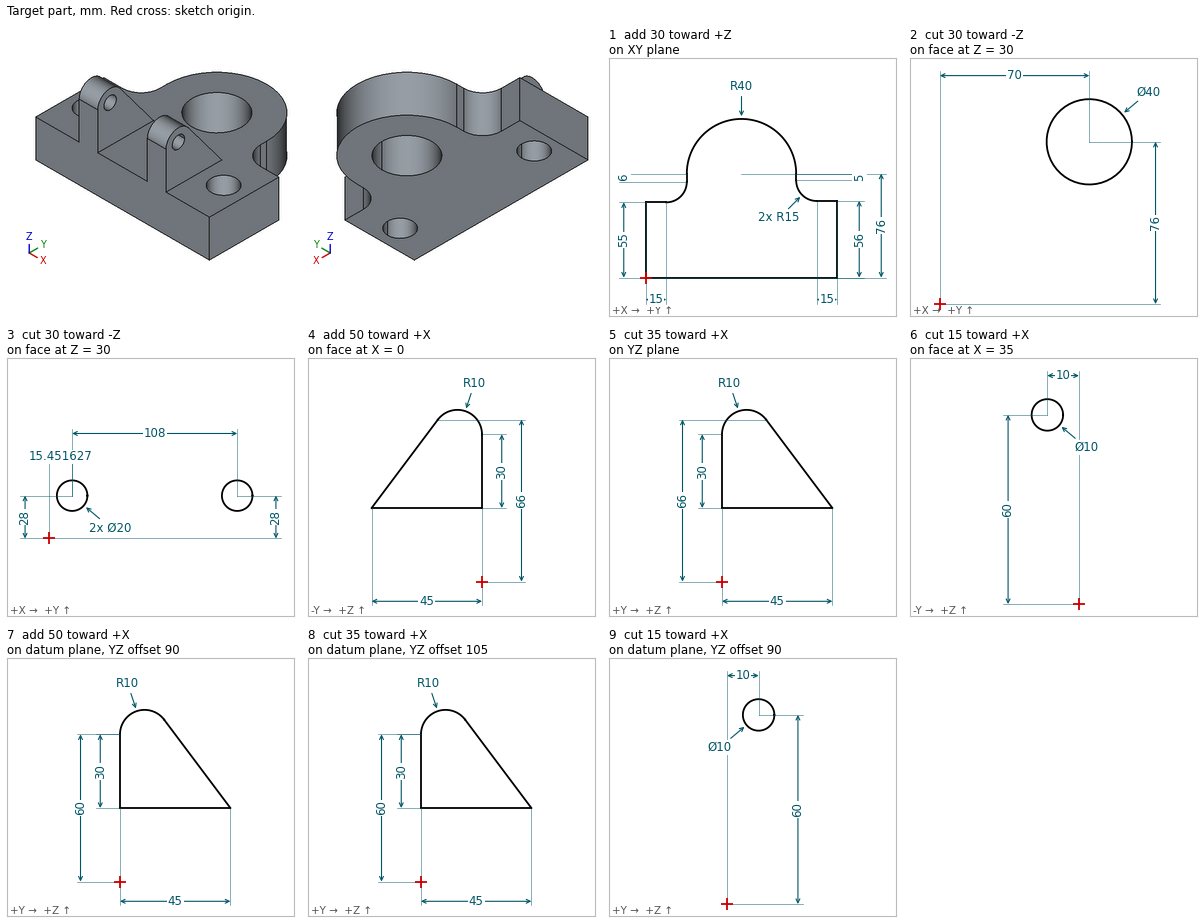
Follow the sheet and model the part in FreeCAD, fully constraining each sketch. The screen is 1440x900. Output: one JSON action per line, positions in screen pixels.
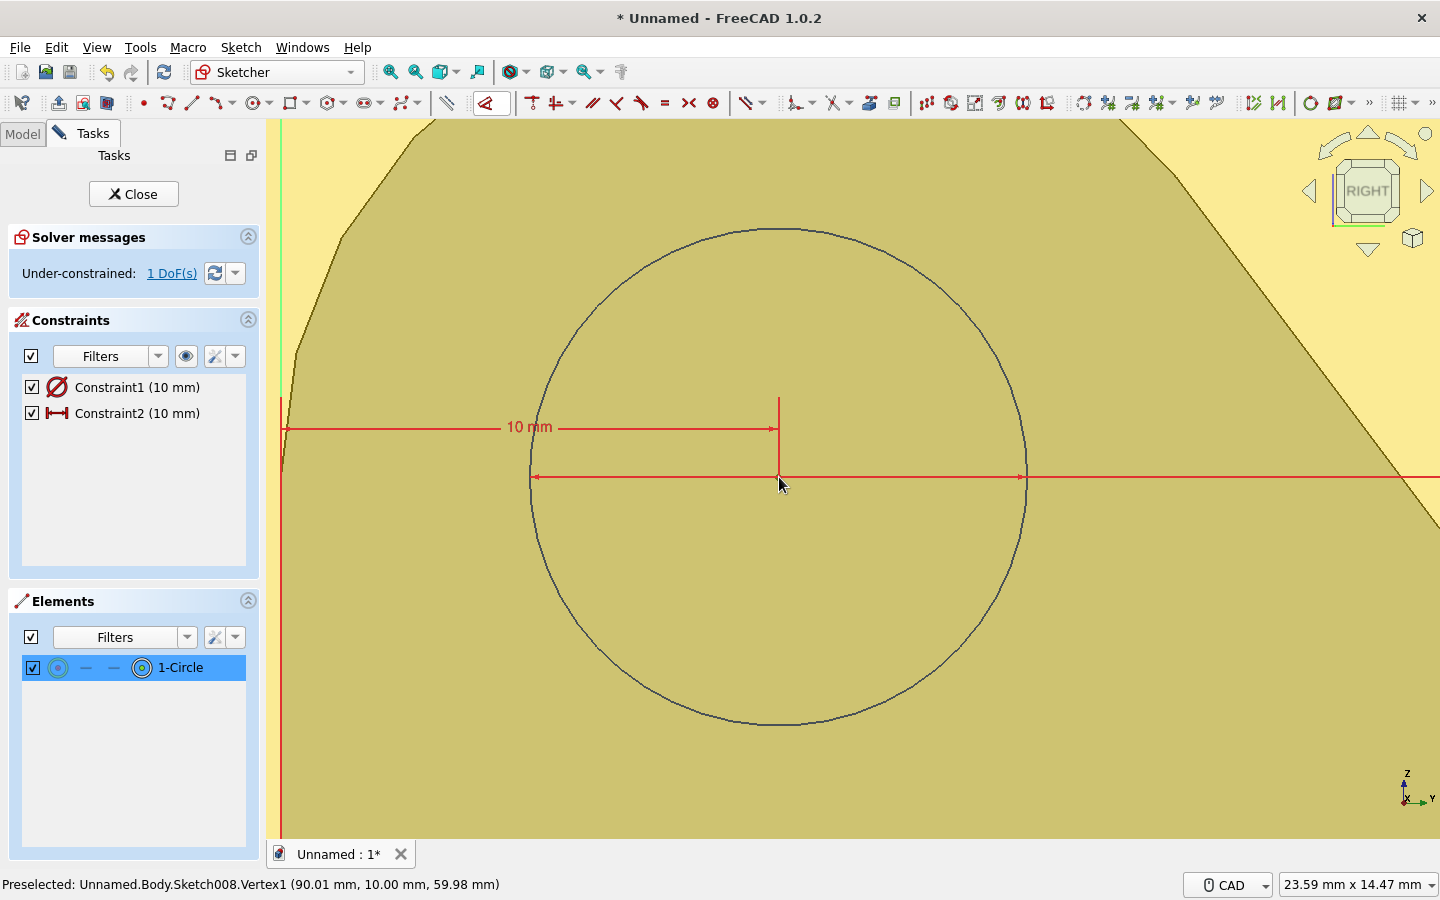
{"action": "key", "text": "i"}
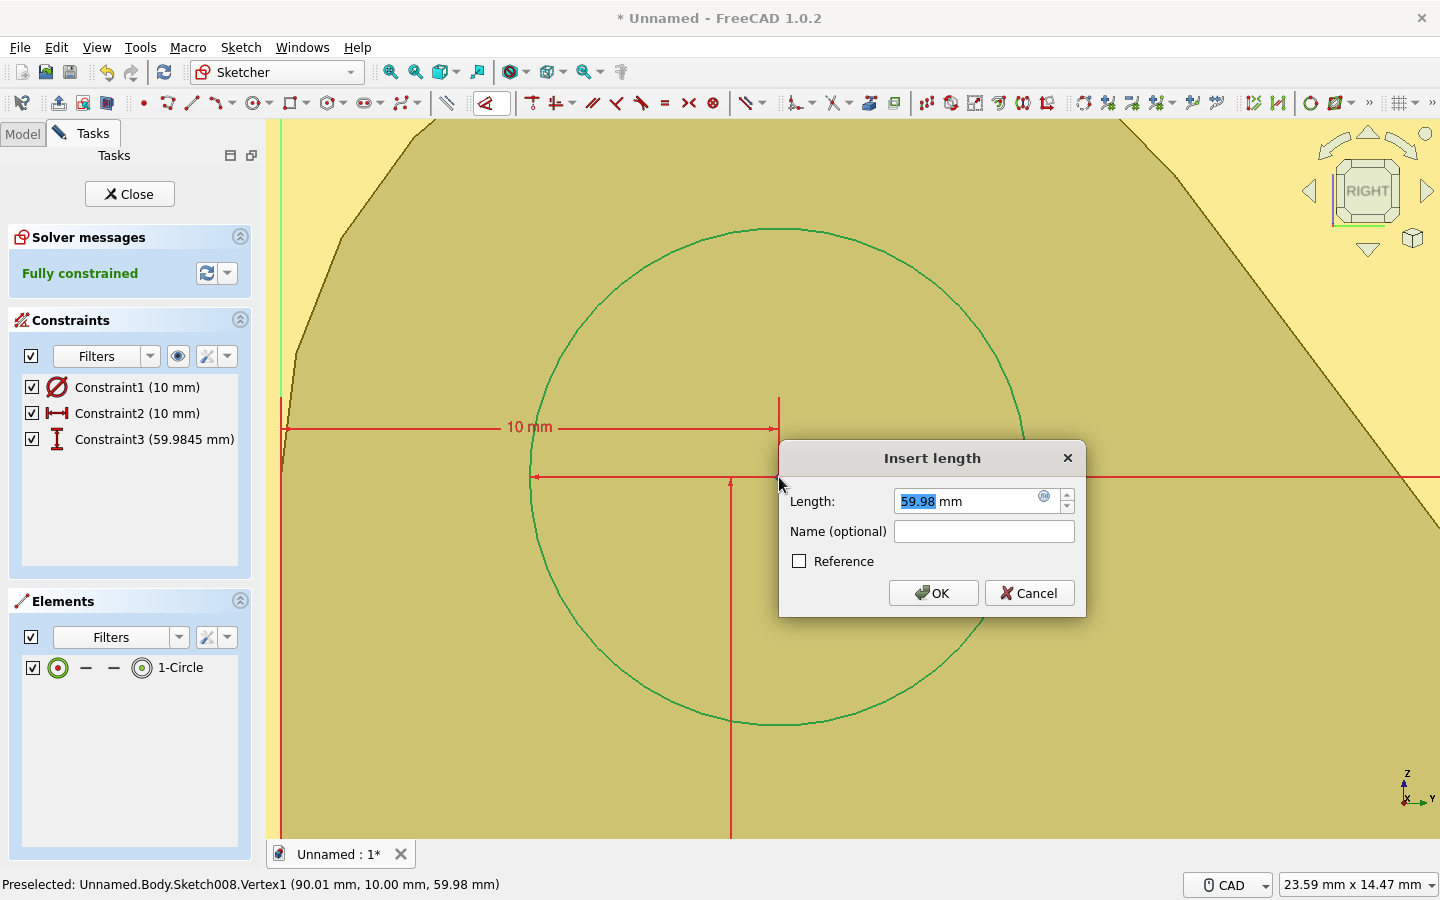
{"action": "type", "text": "60"}
{"action": "key", "text": "Return"}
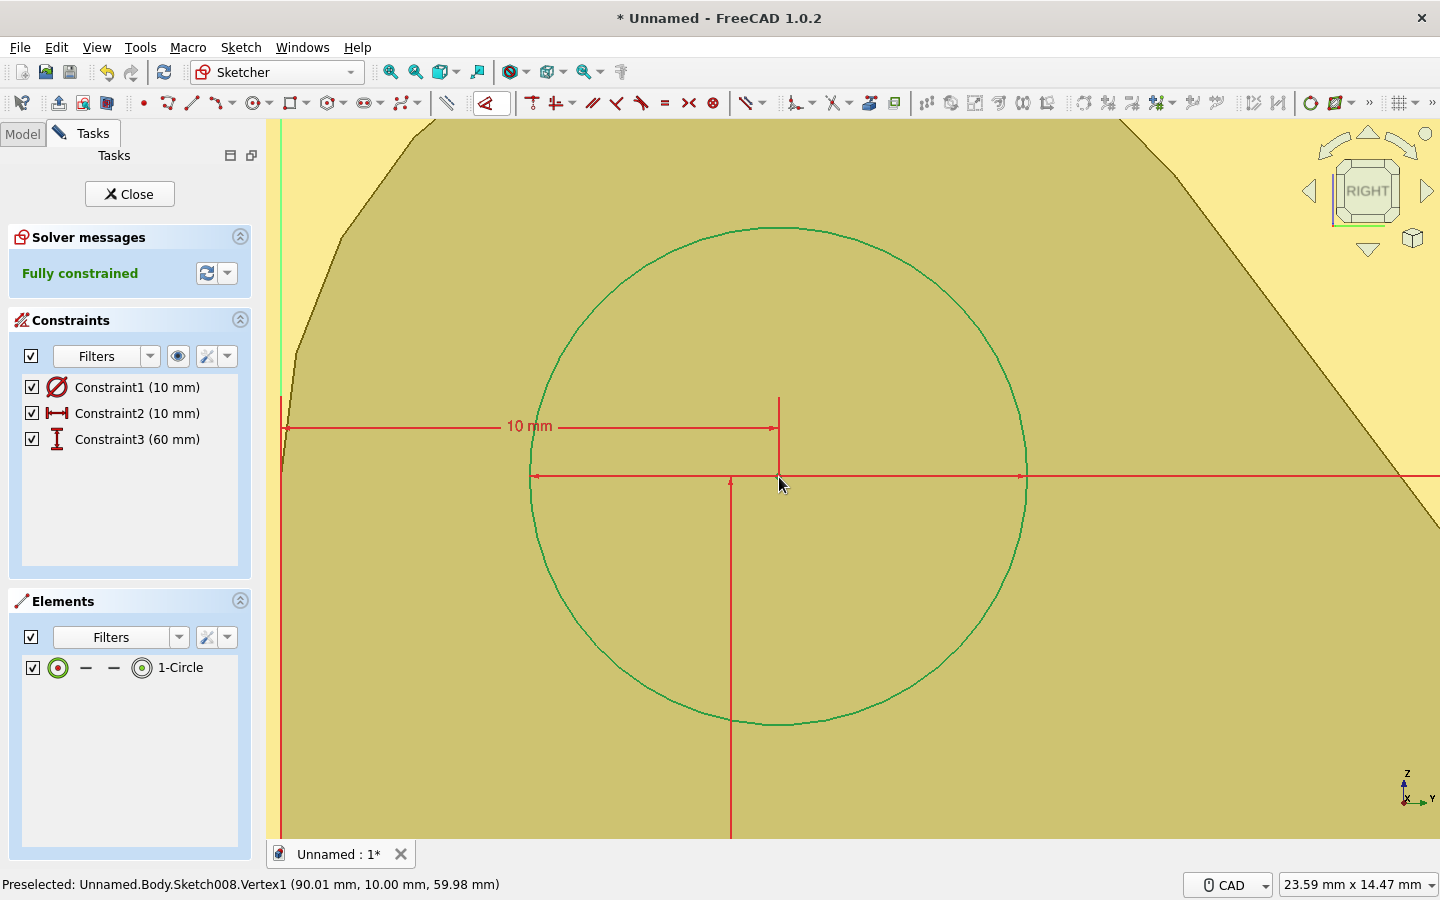
{"action": "left_click", "coordinate": [130, 194]}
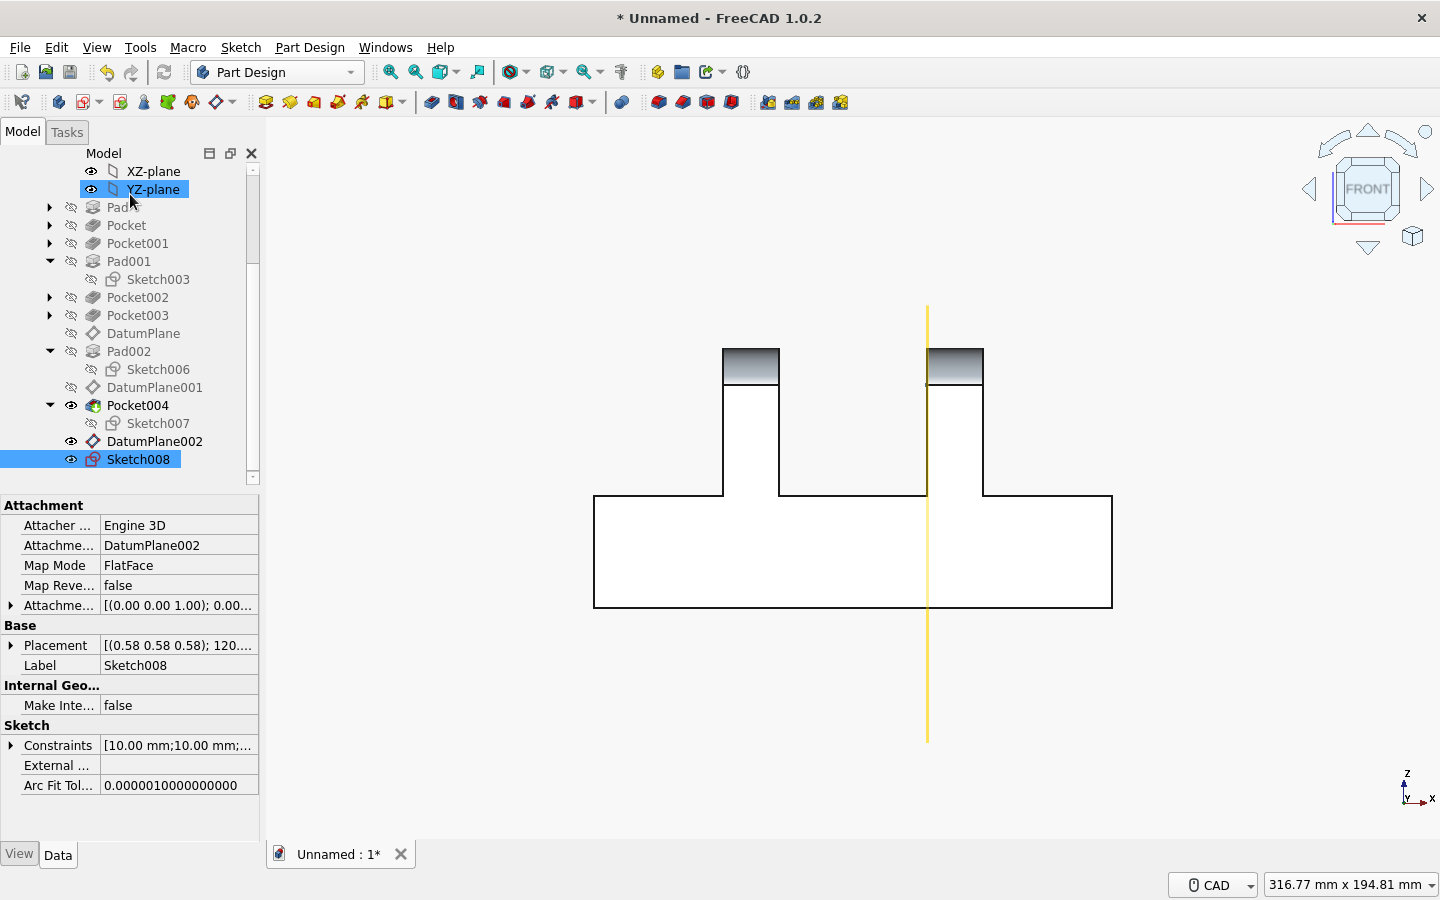
{"action": "left_click", "coordinate": [432, 102]}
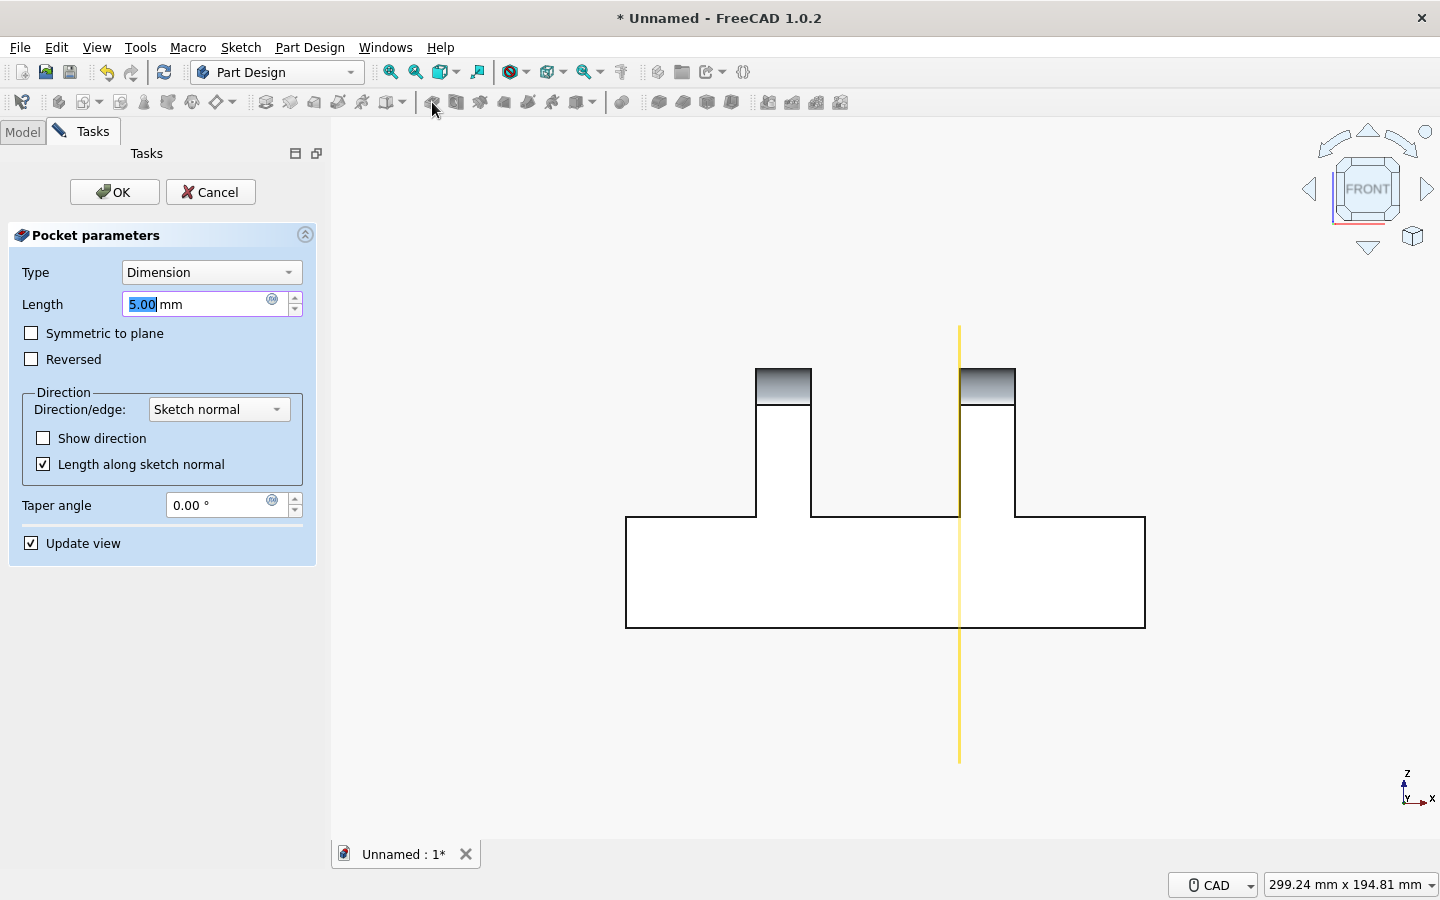
{"action": "type", "text": "15"}
{"action": "key", "text": "Tab"}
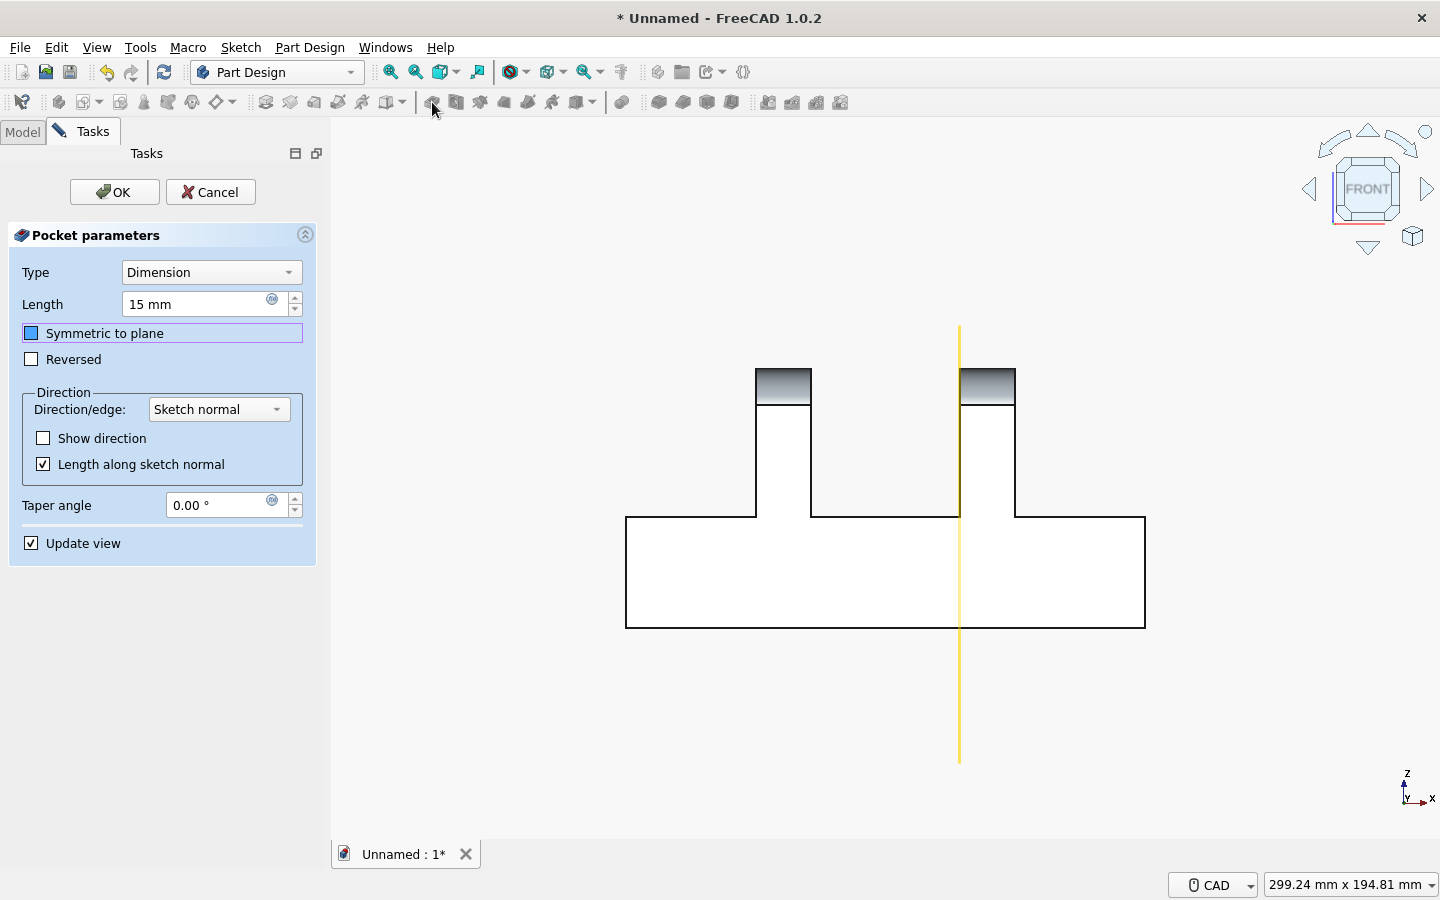
{"action": "left_click", "coordinate": [30, 359]}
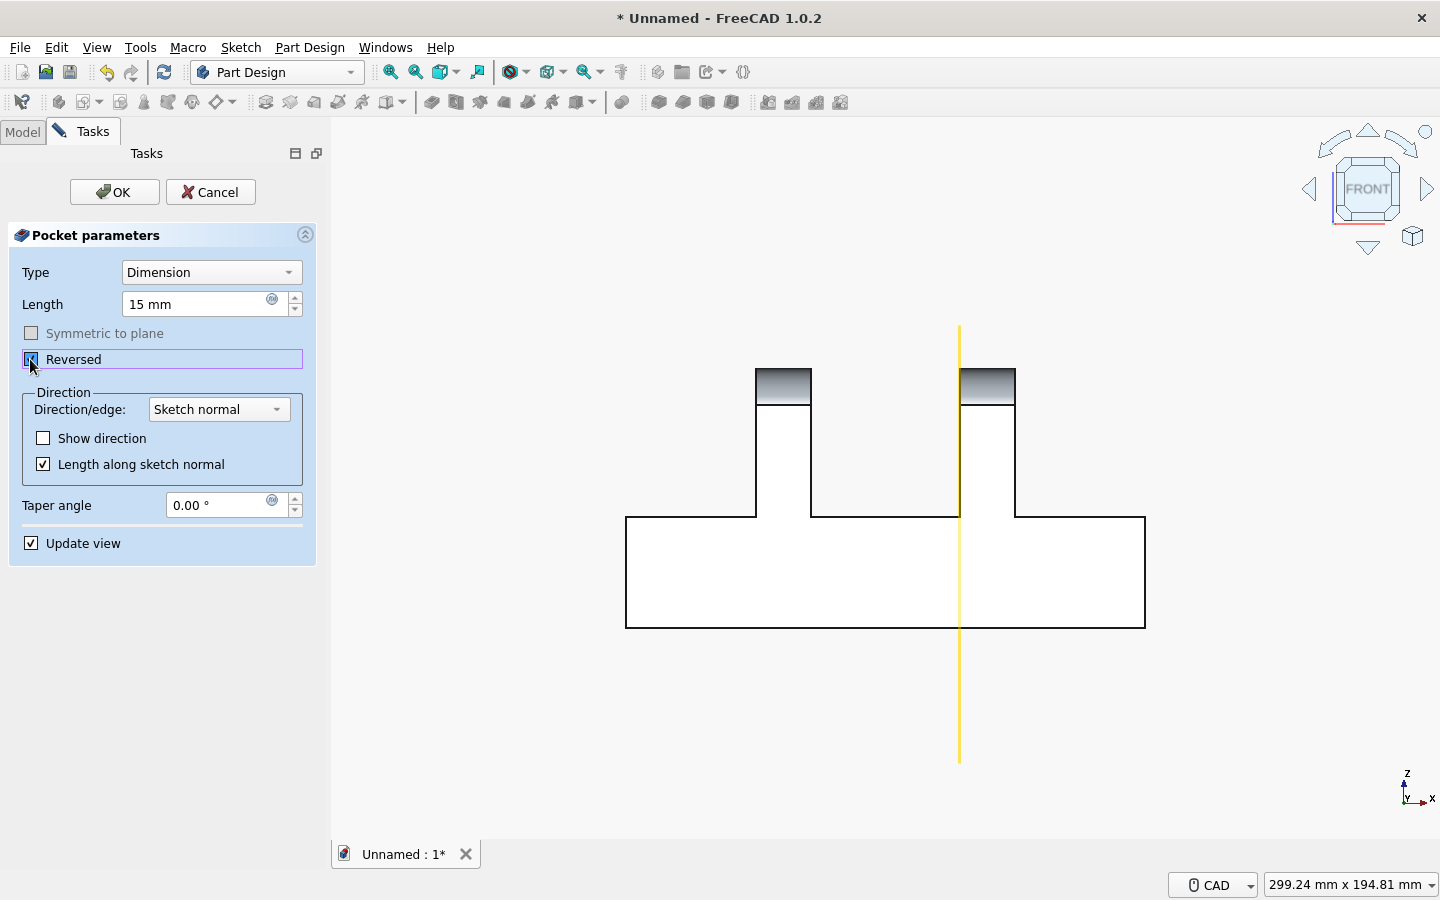
{"action": "left_click", "coordinate": [115, 192]}